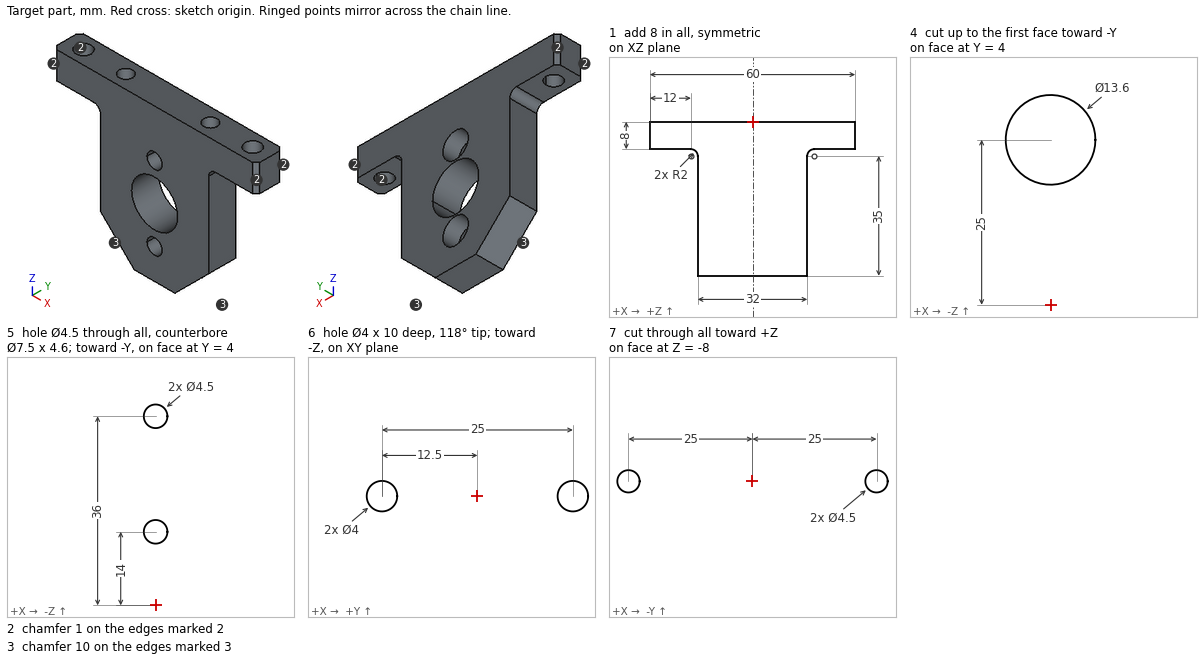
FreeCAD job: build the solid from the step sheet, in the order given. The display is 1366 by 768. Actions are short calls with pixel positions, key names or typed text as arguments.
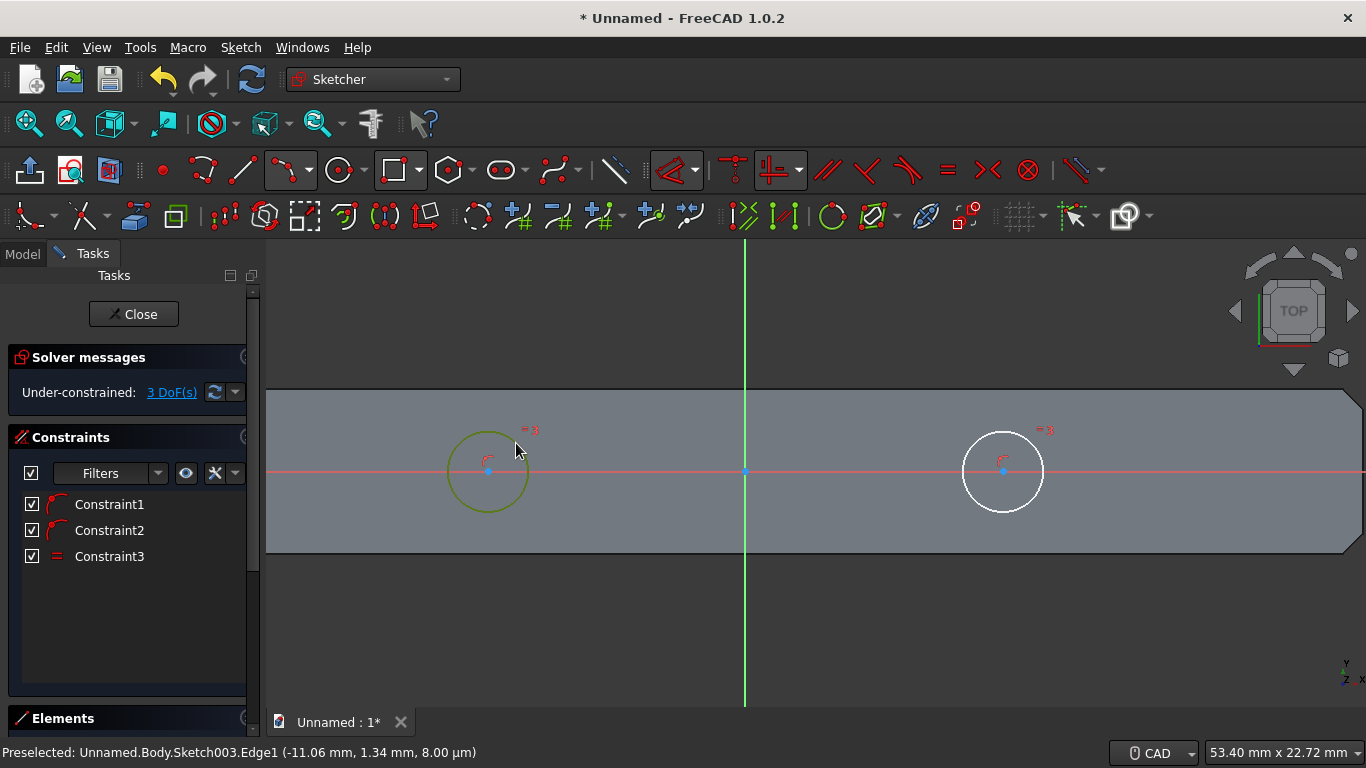
key(k)
key(o)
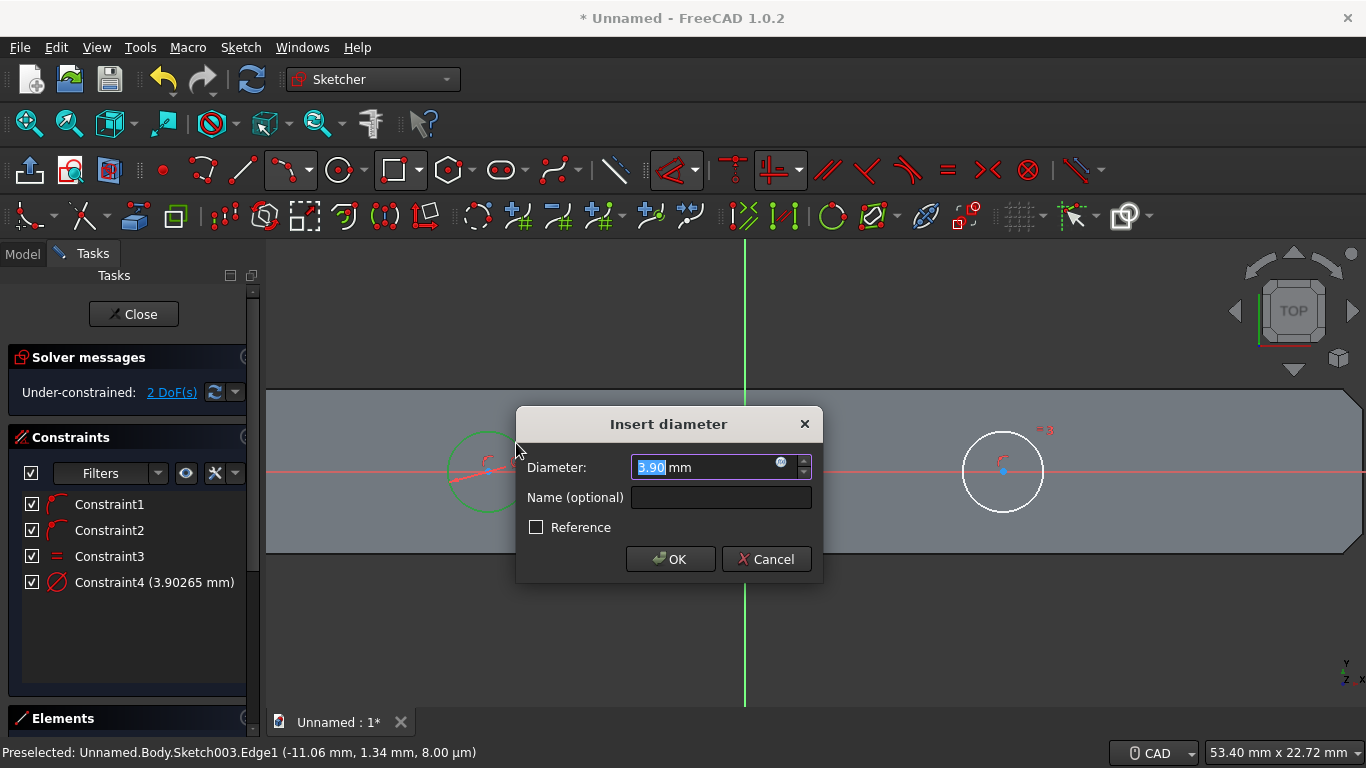
text(4)
key(Return)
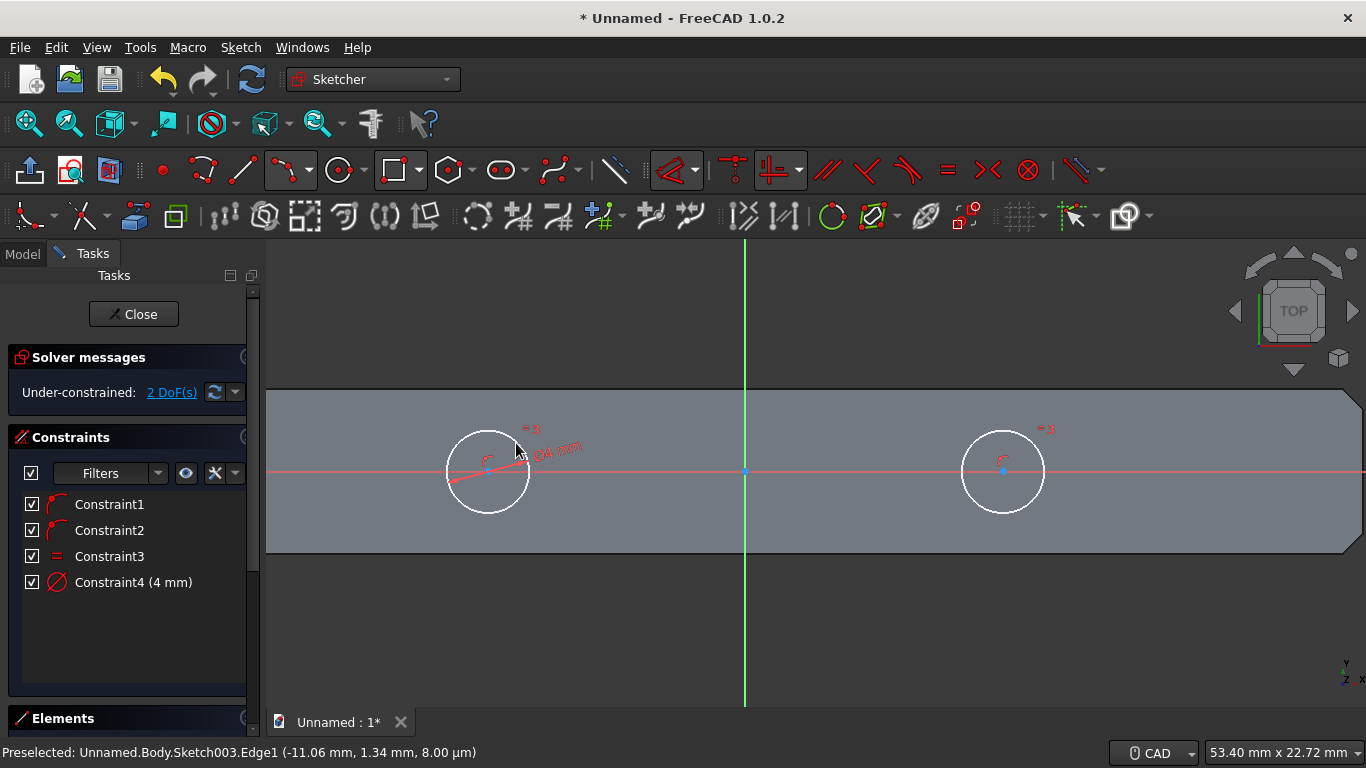
click(488, 472)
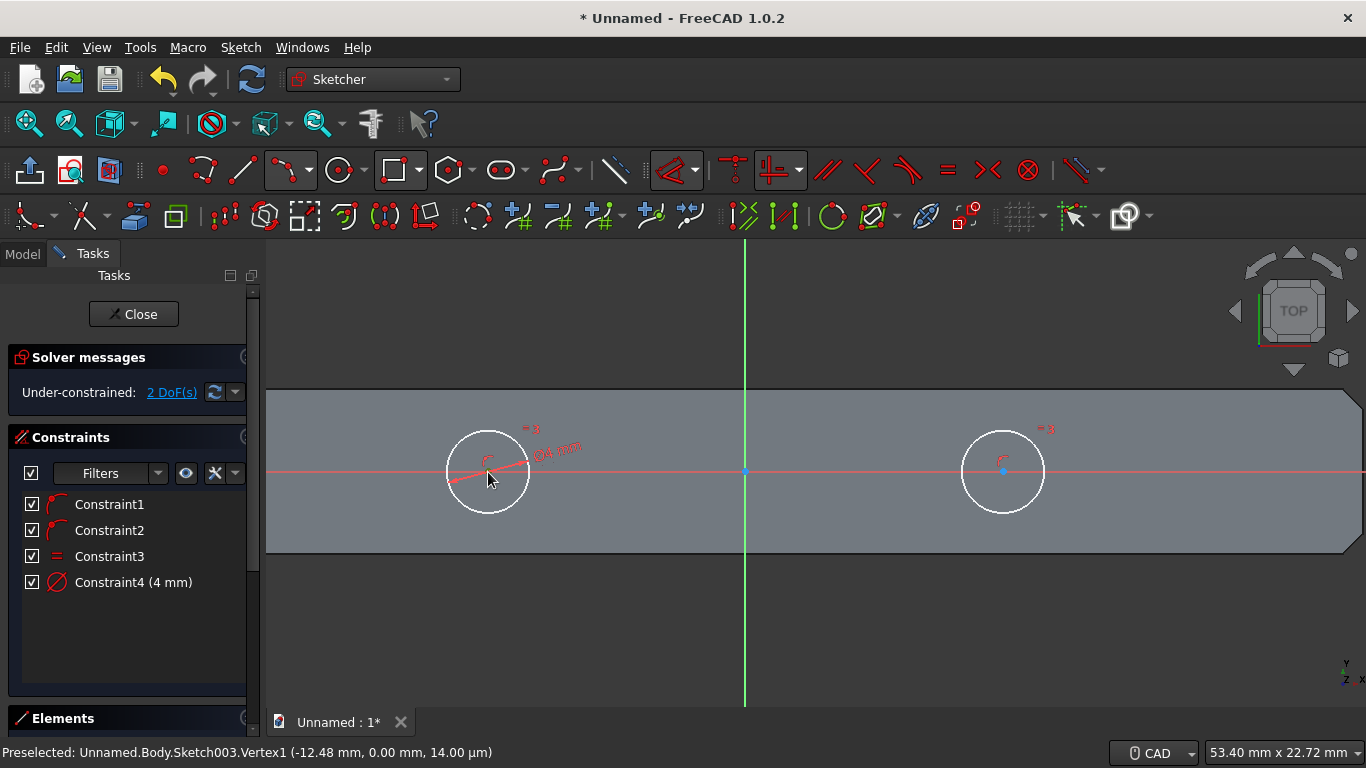
click(1003, 472)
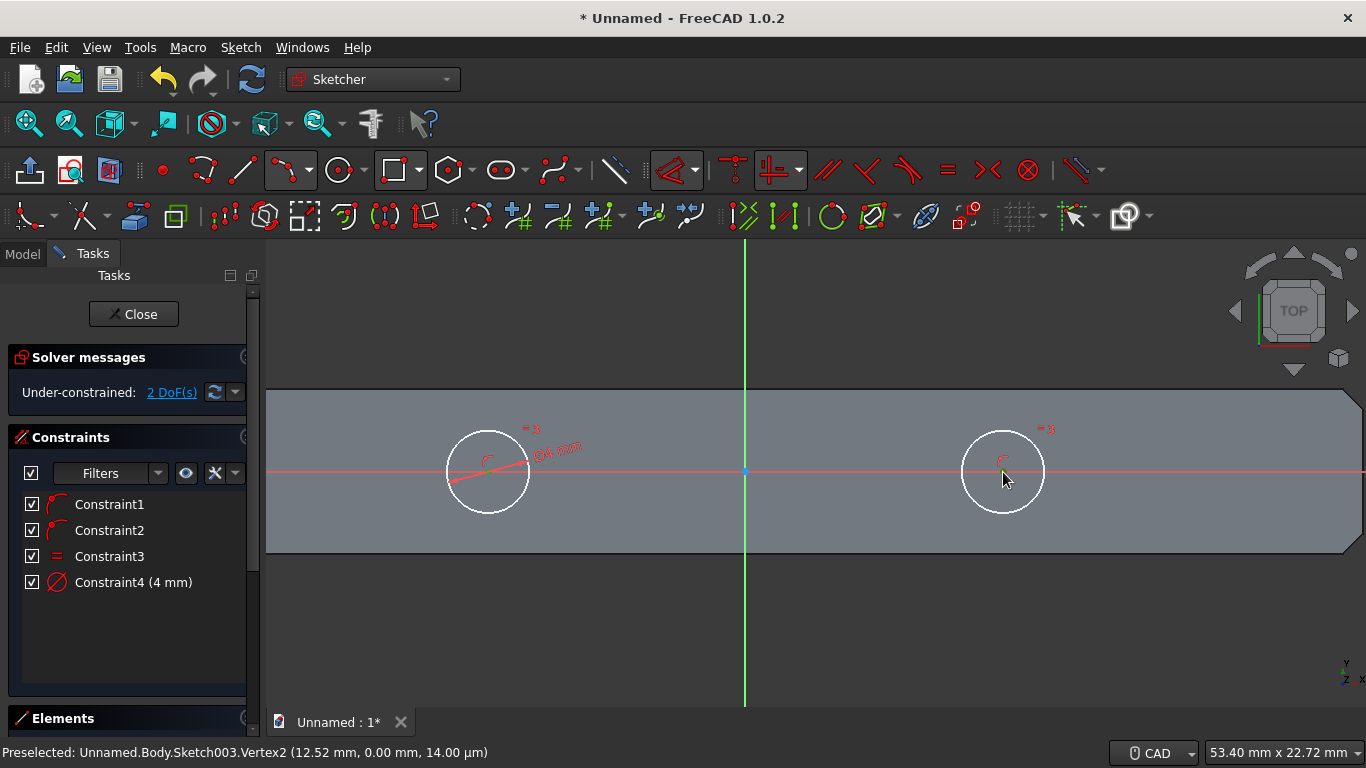
key(l)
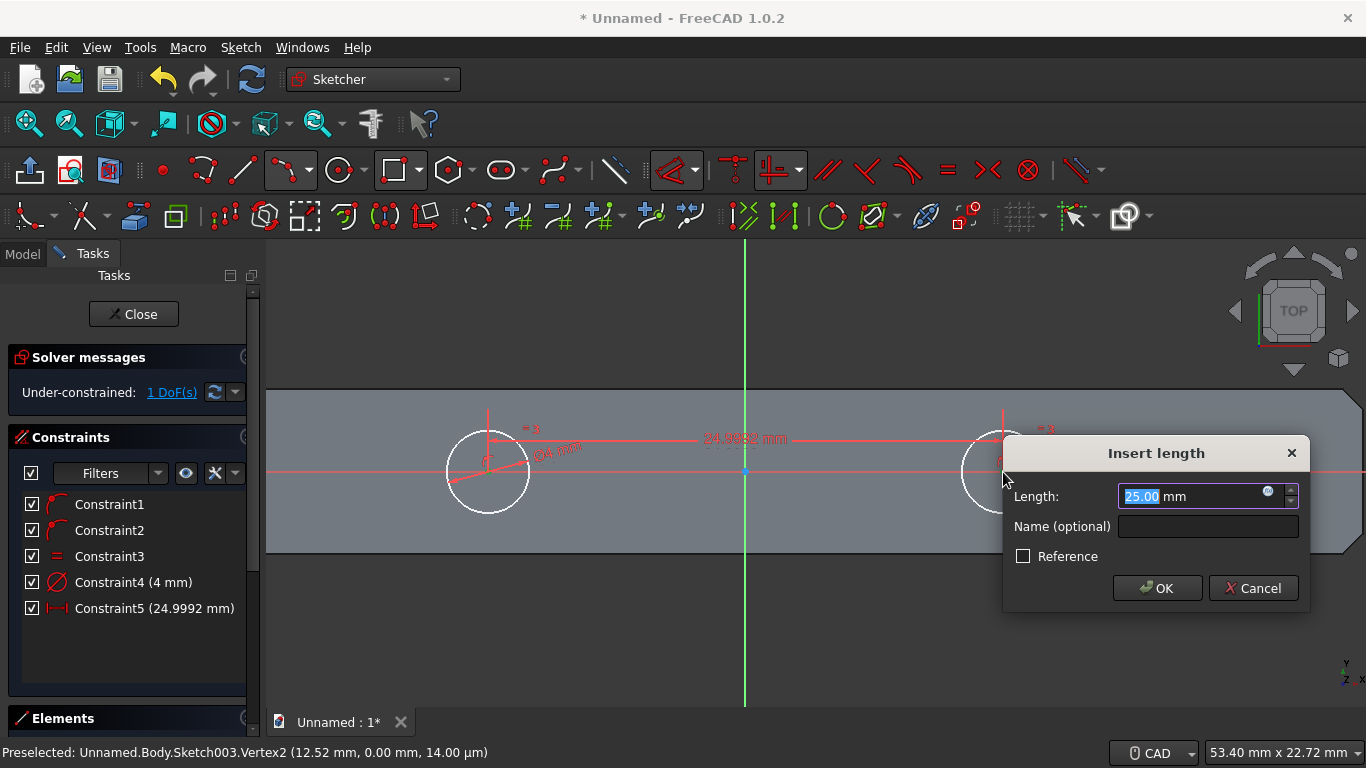
text(25)
key(Return)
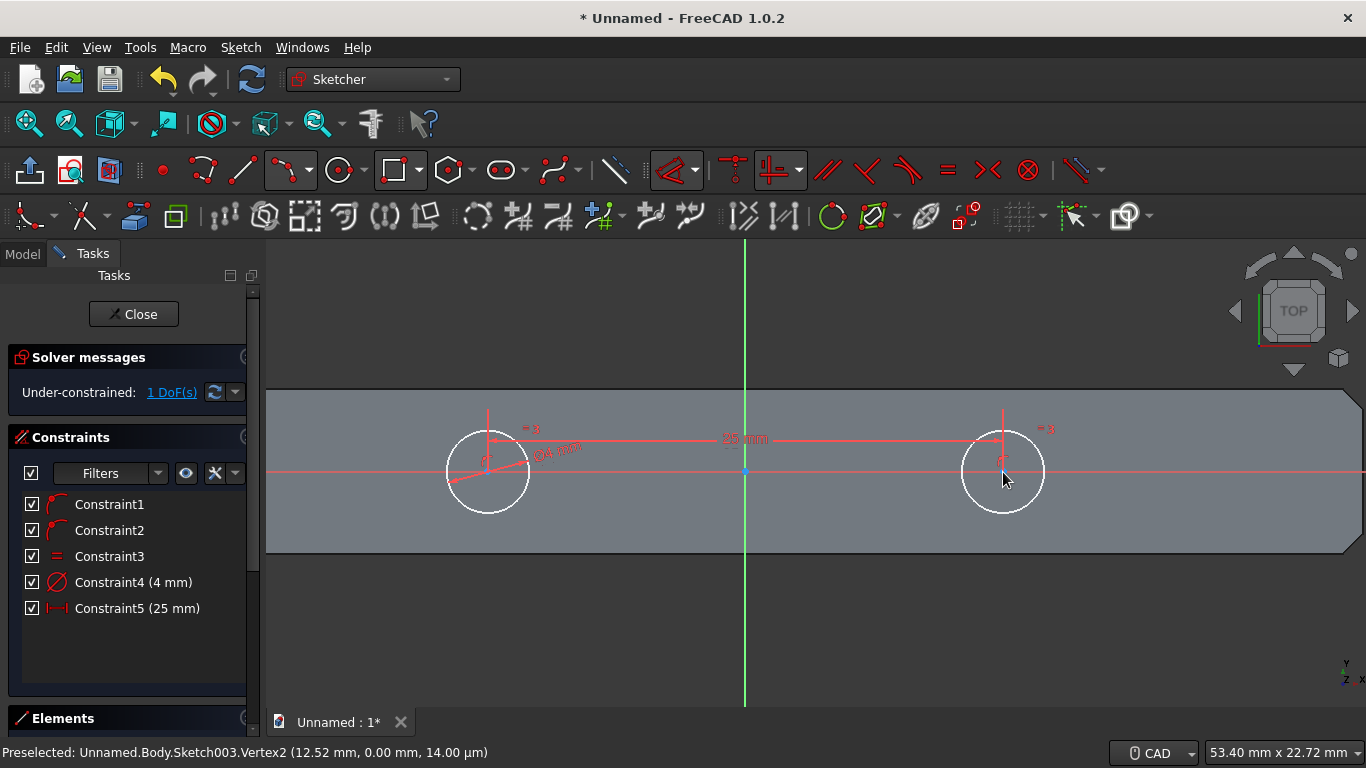
click(488, 472)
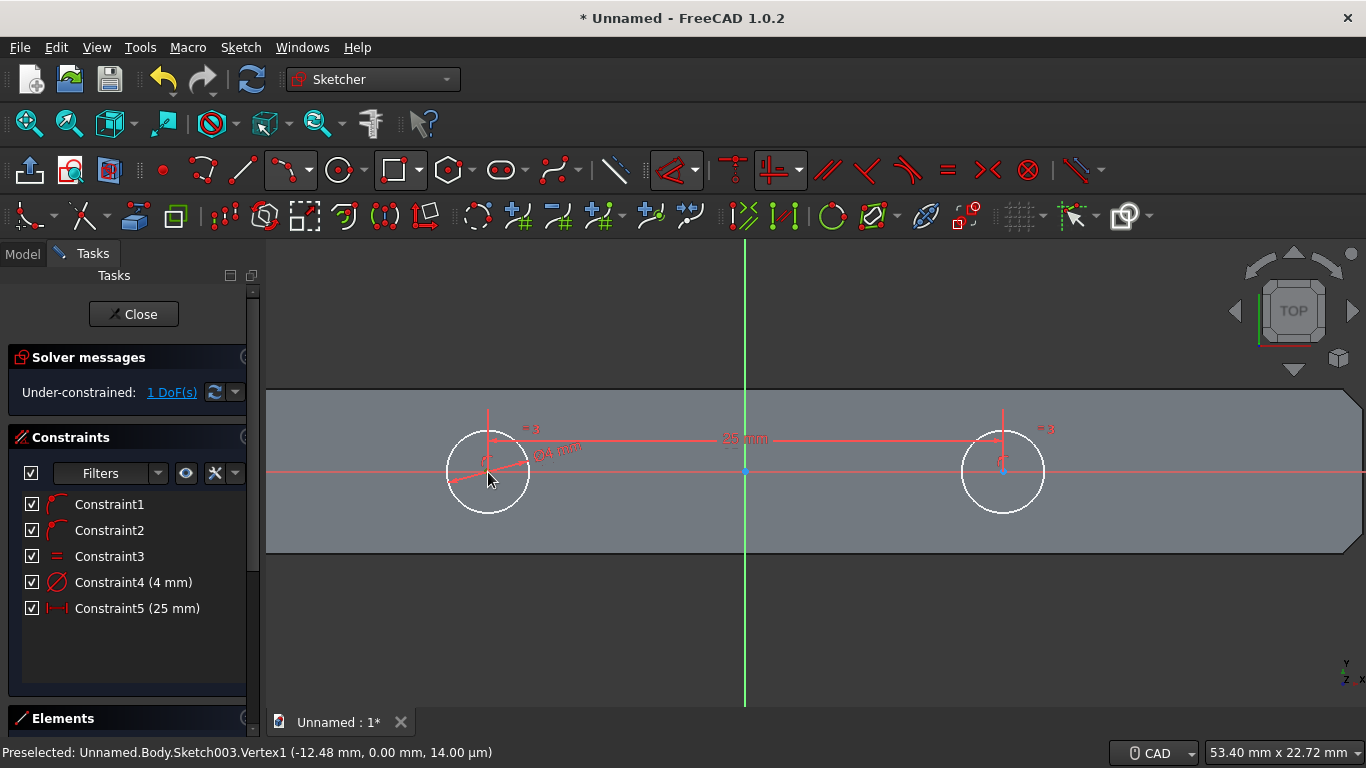
click(698, 170)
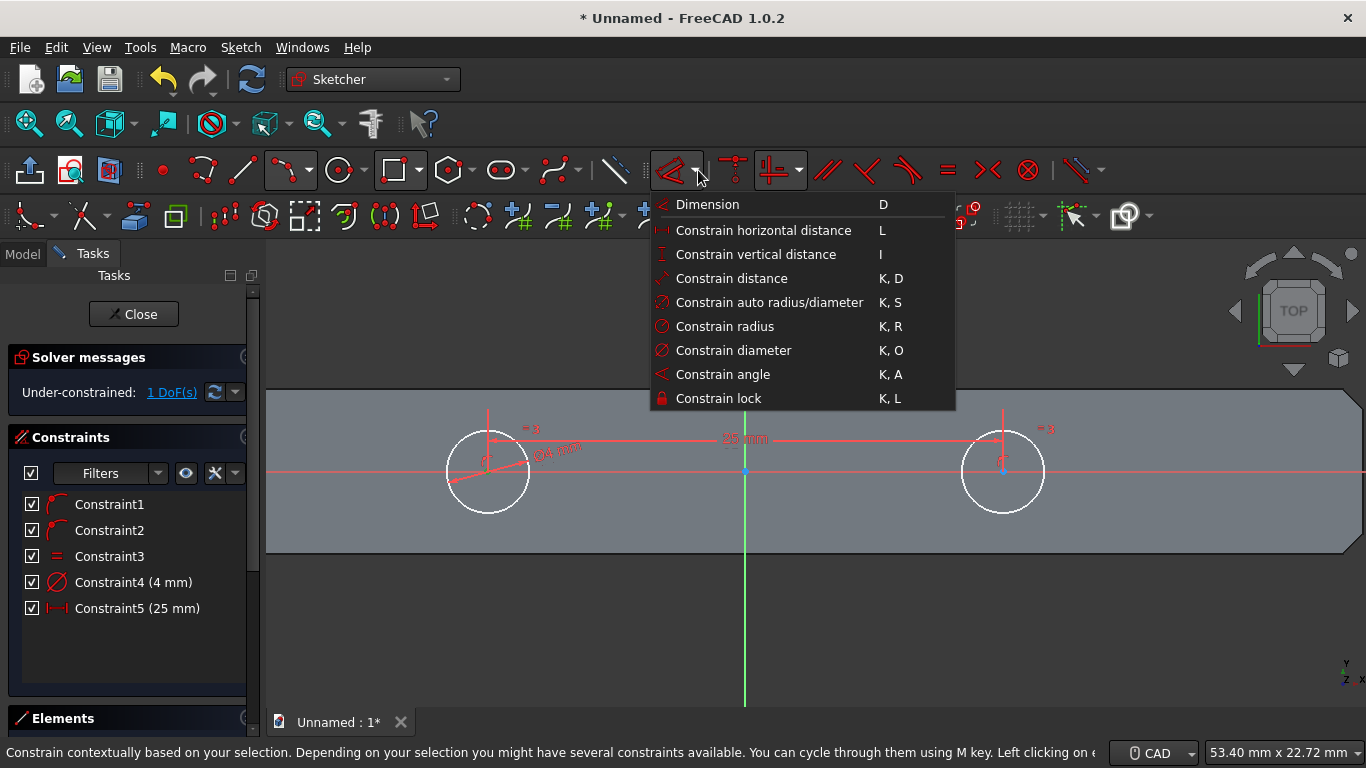
click(803, 230)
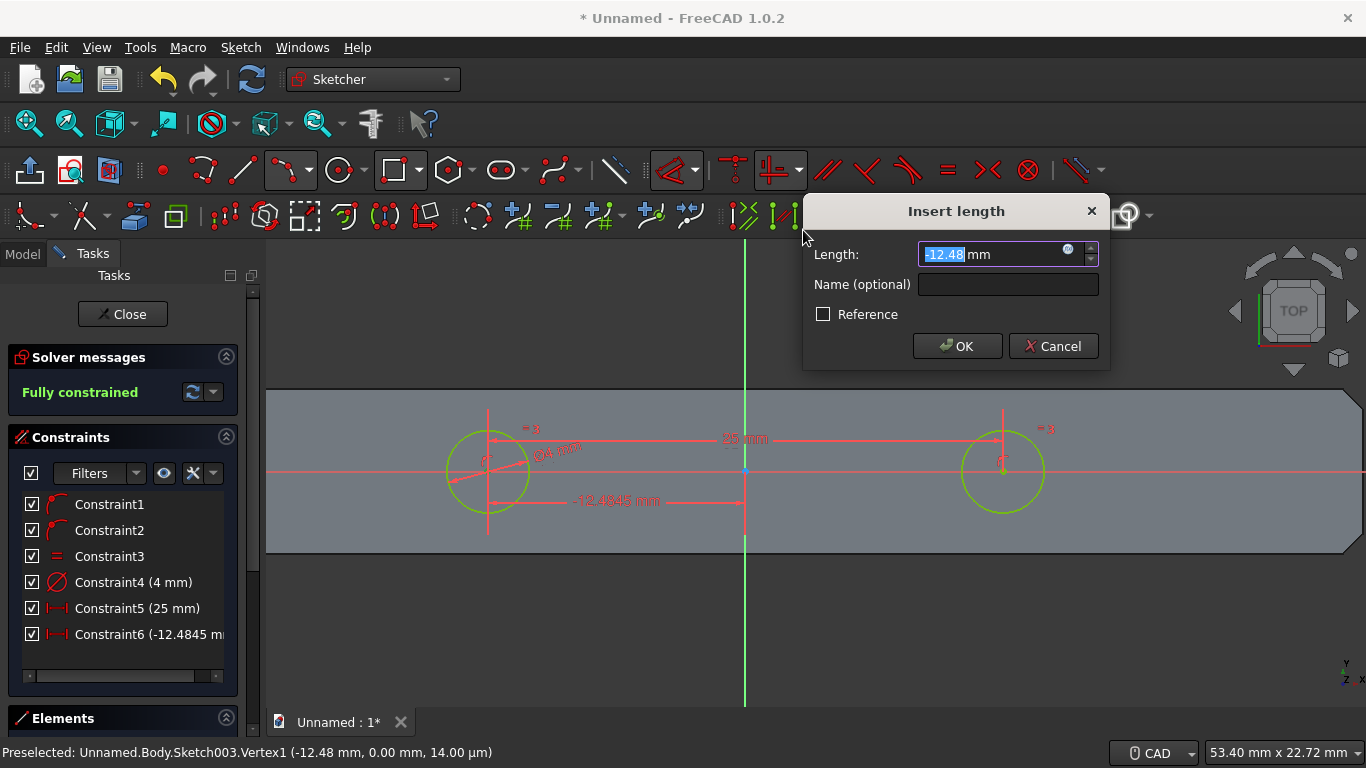
text(-12.5)
key(Return)